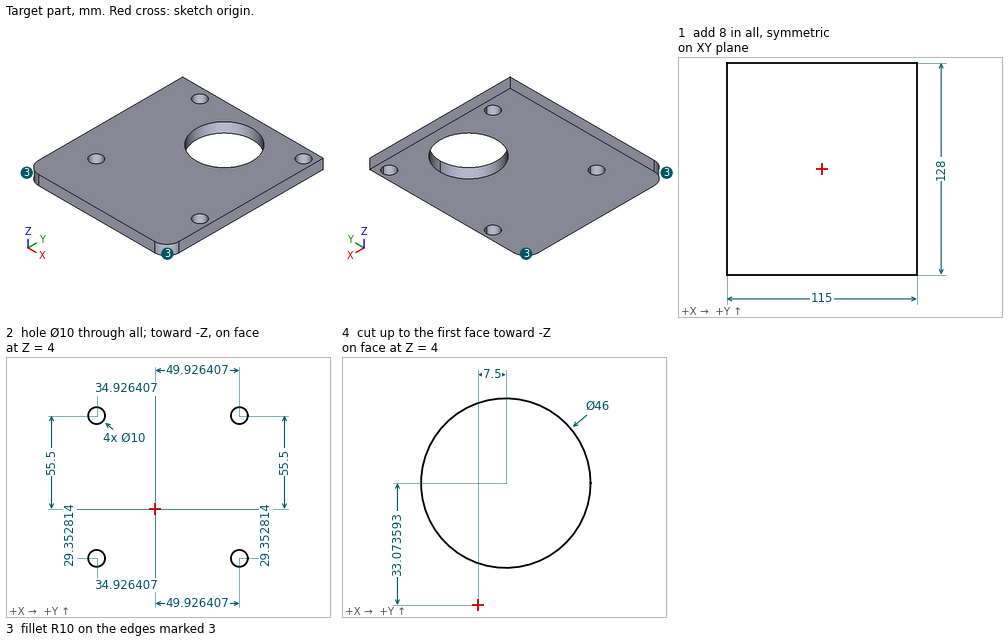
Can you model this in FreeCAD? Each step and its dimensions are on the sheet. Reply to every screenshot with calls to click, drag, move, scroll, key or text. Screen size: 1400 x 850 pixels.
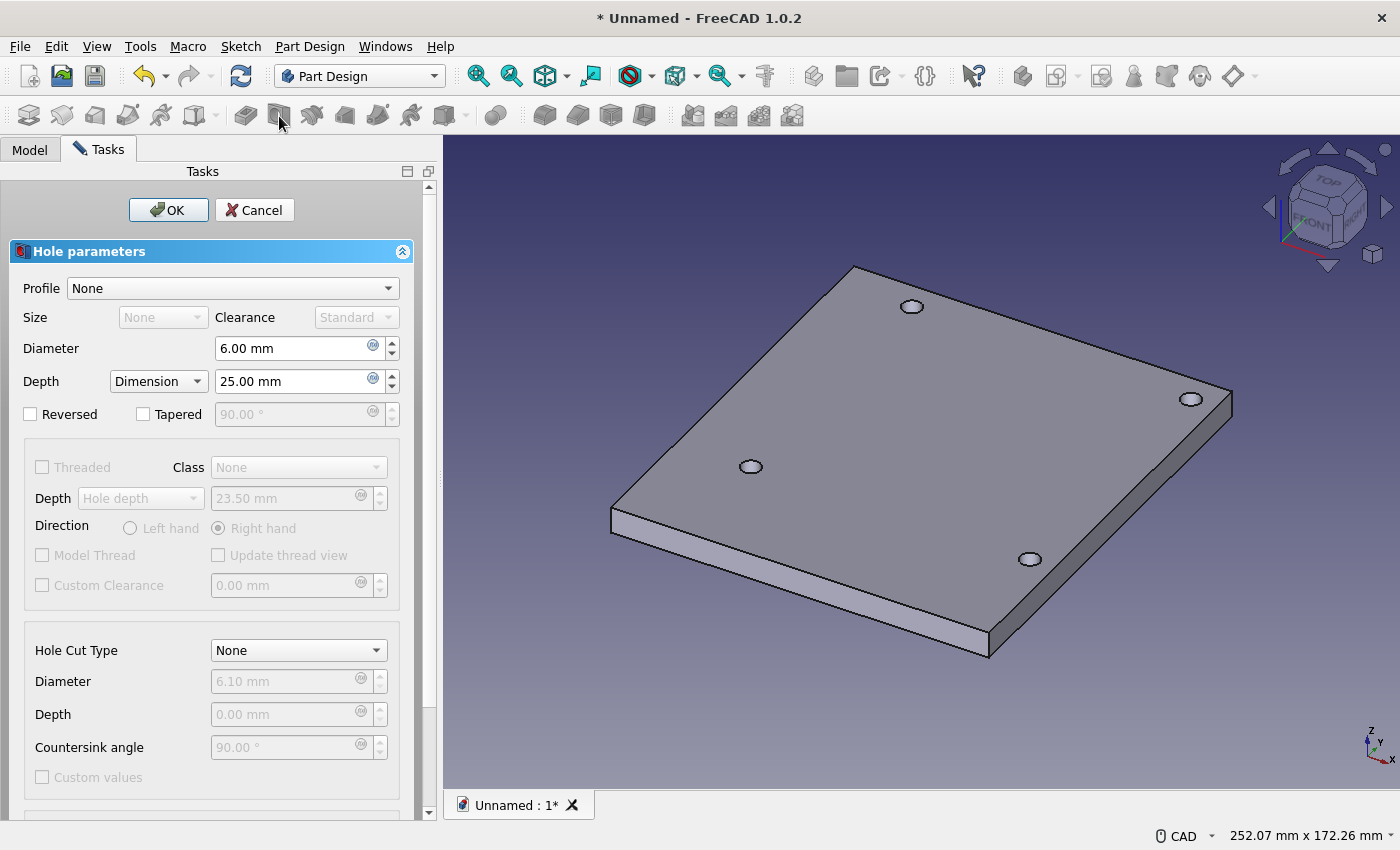
triple_click(300, 348)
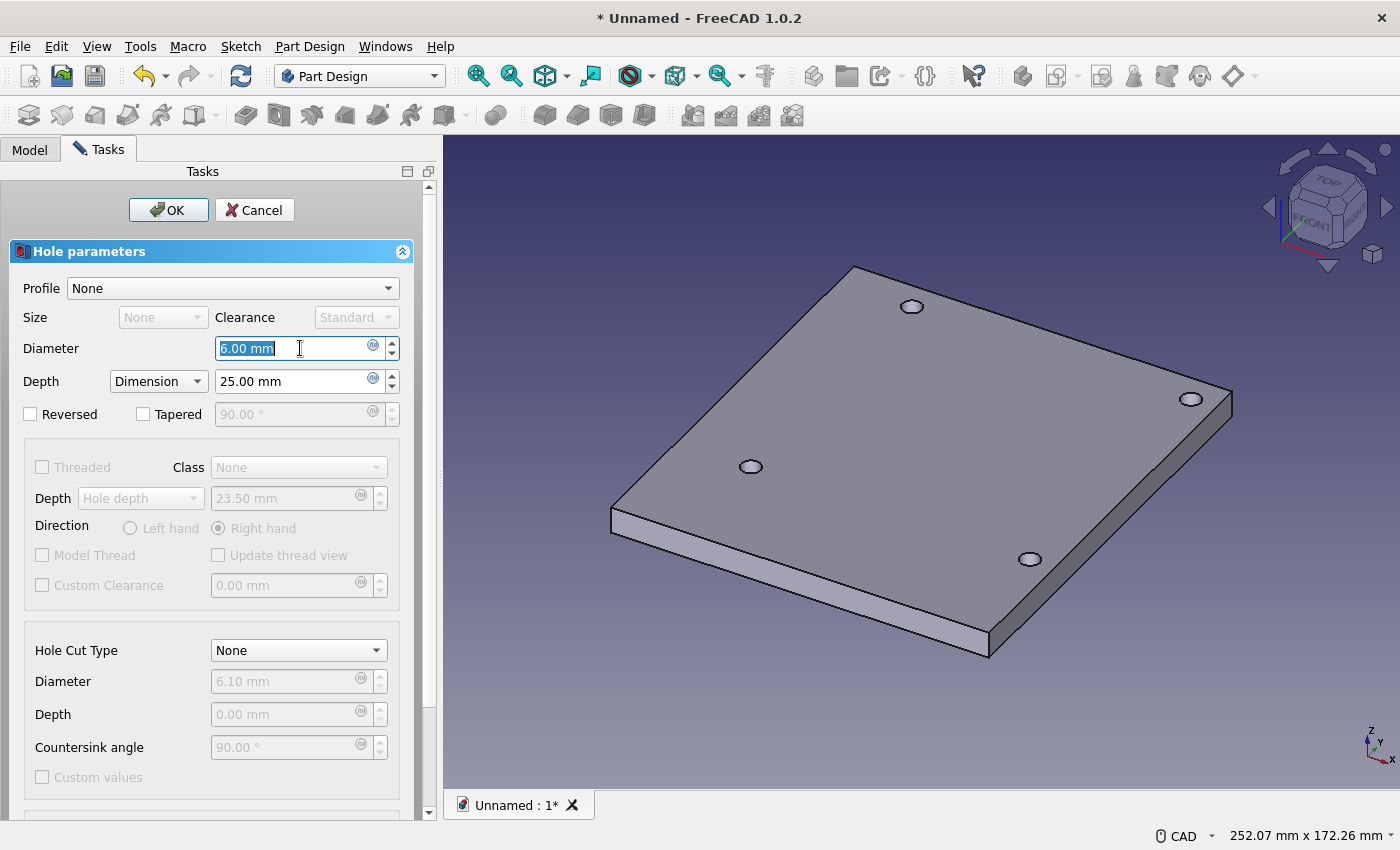
text(10)
key(Tab)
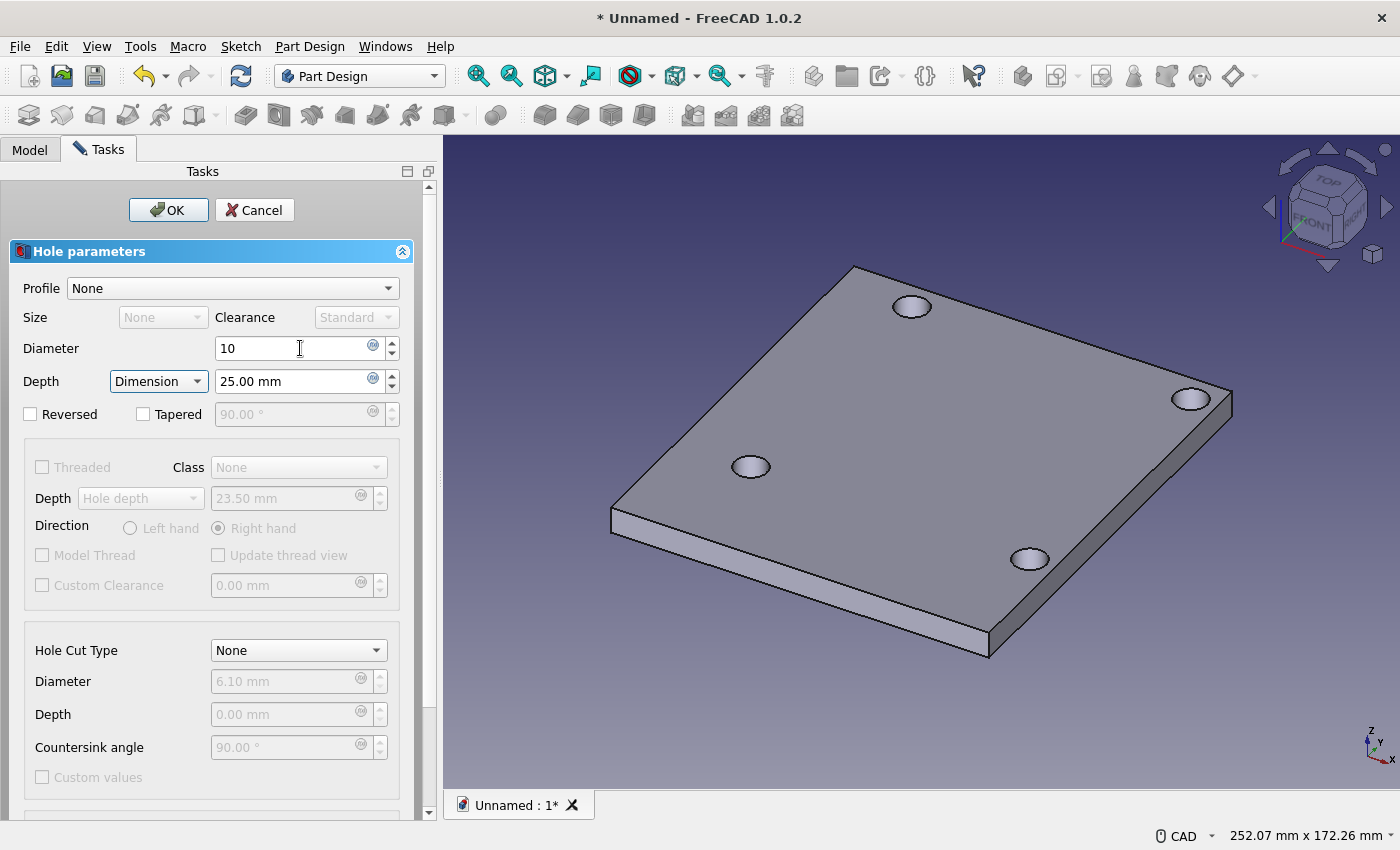
click(160, 382)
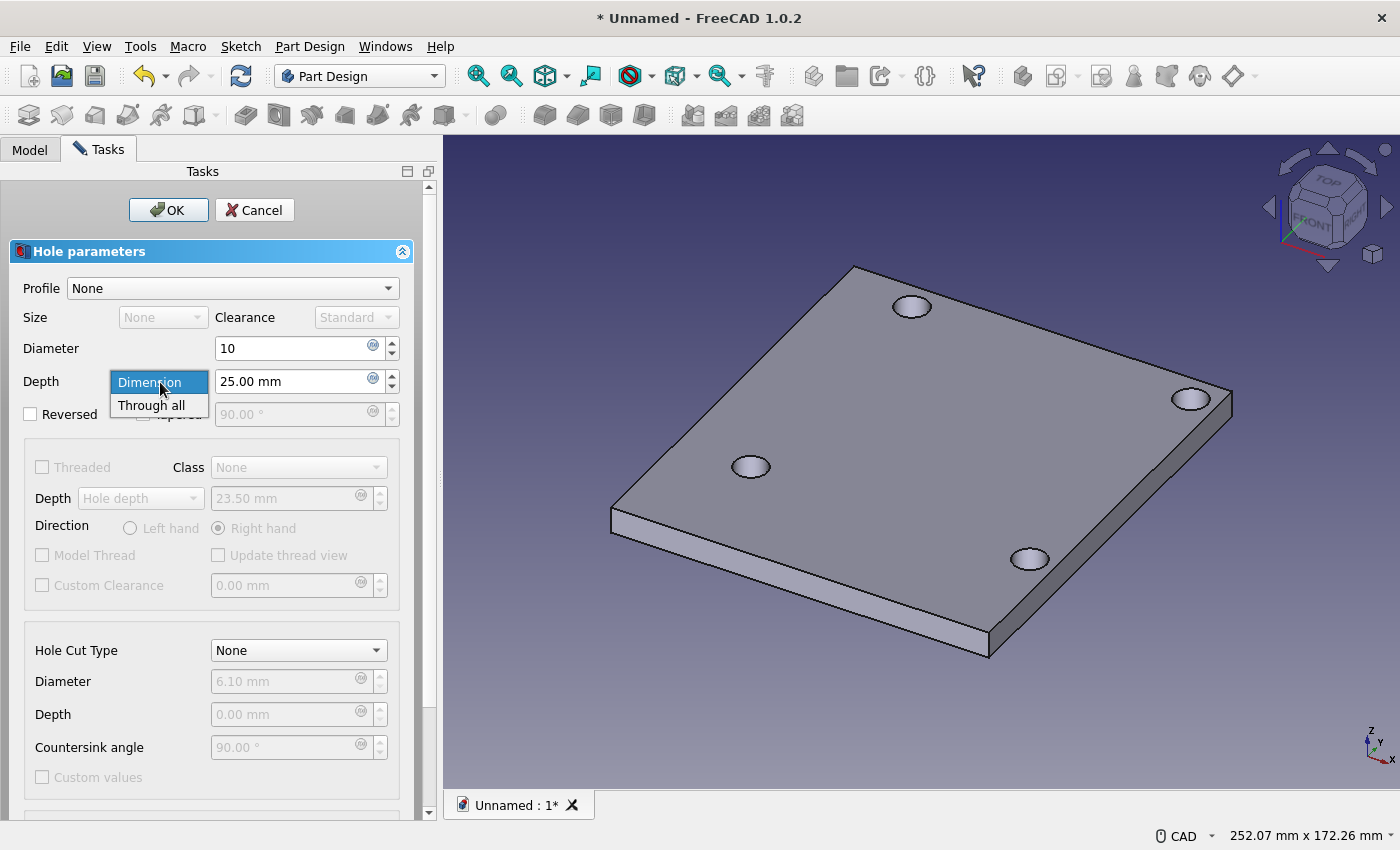
click(158, 406)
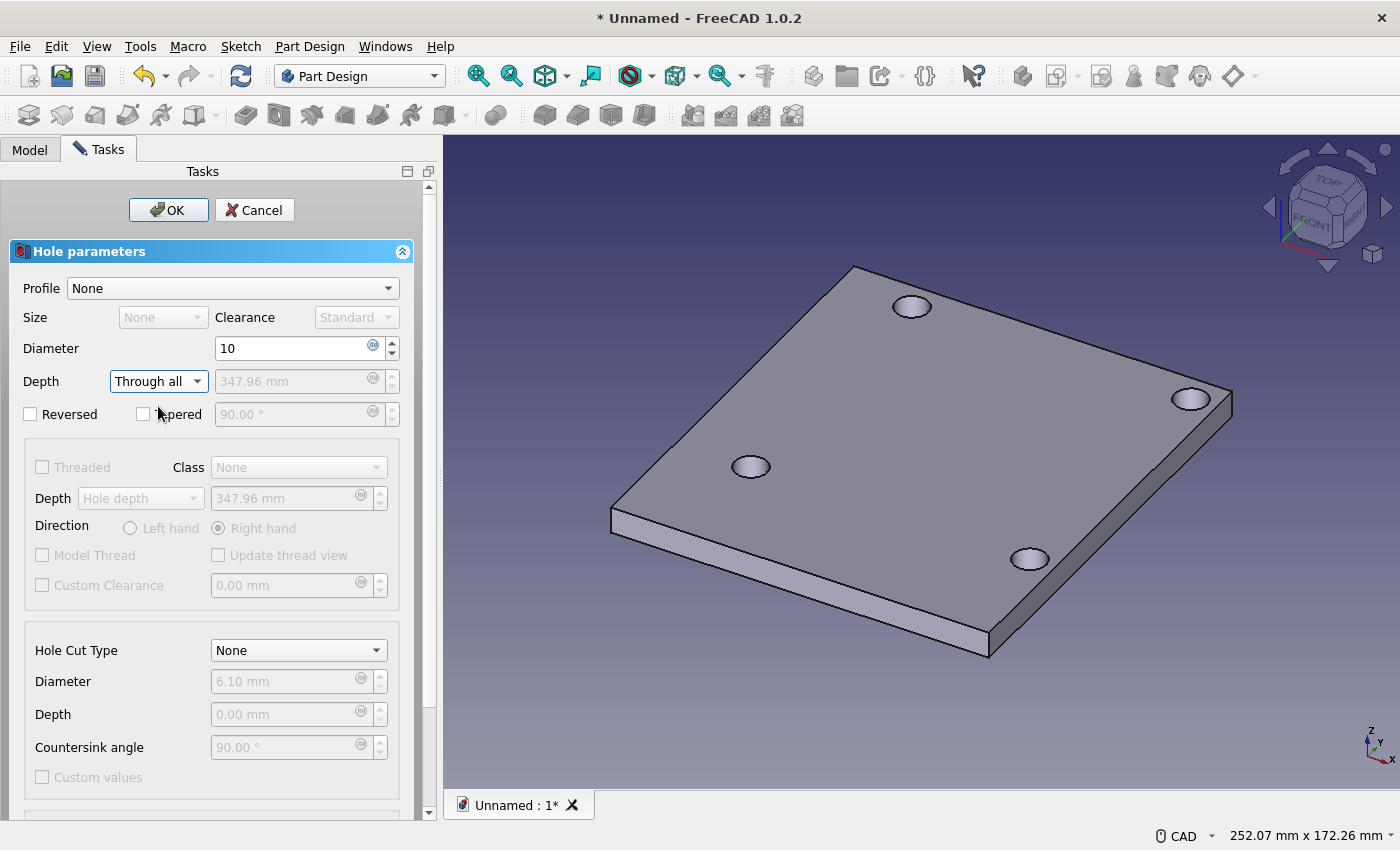
click(169, 210)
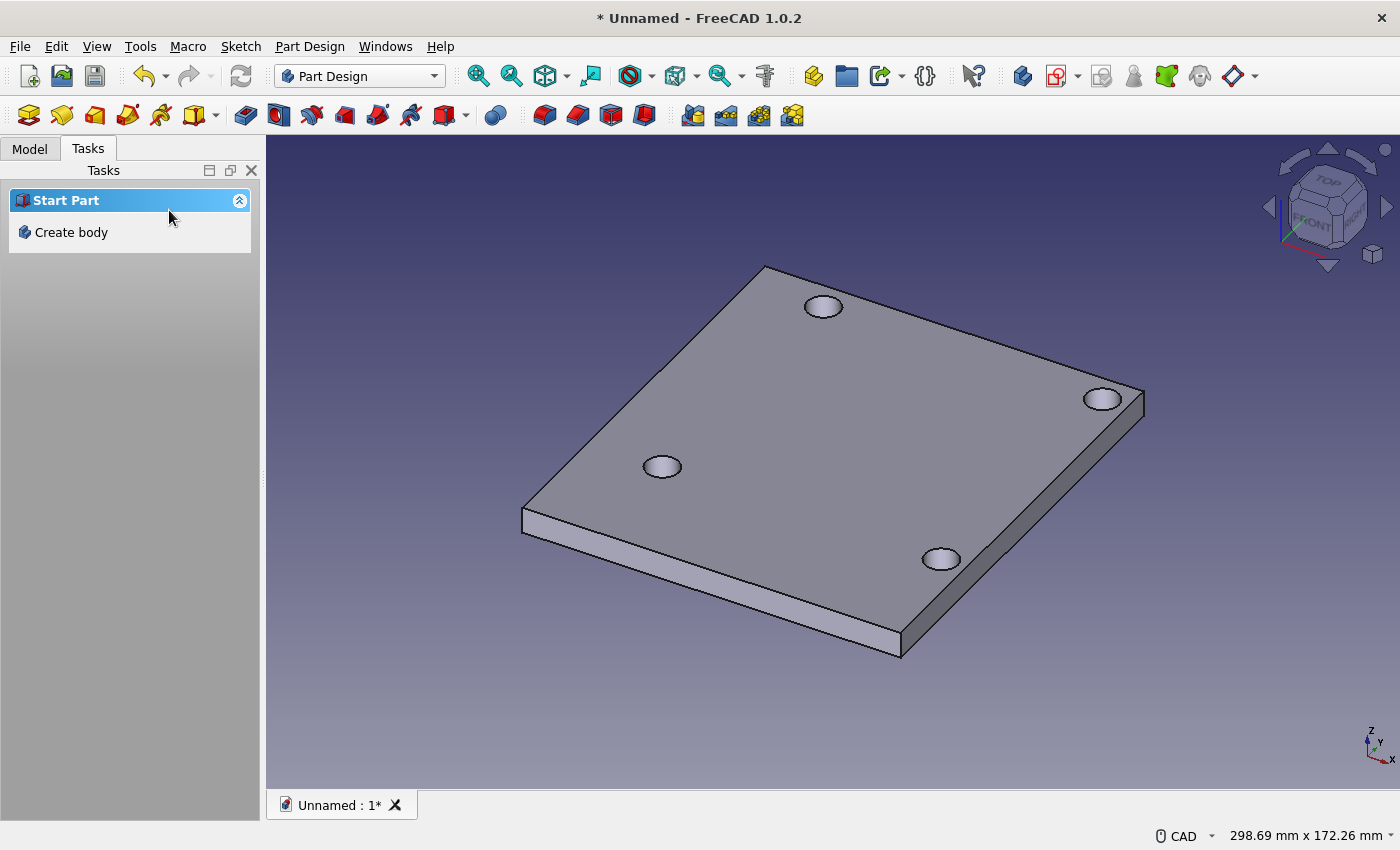
click(901, 644)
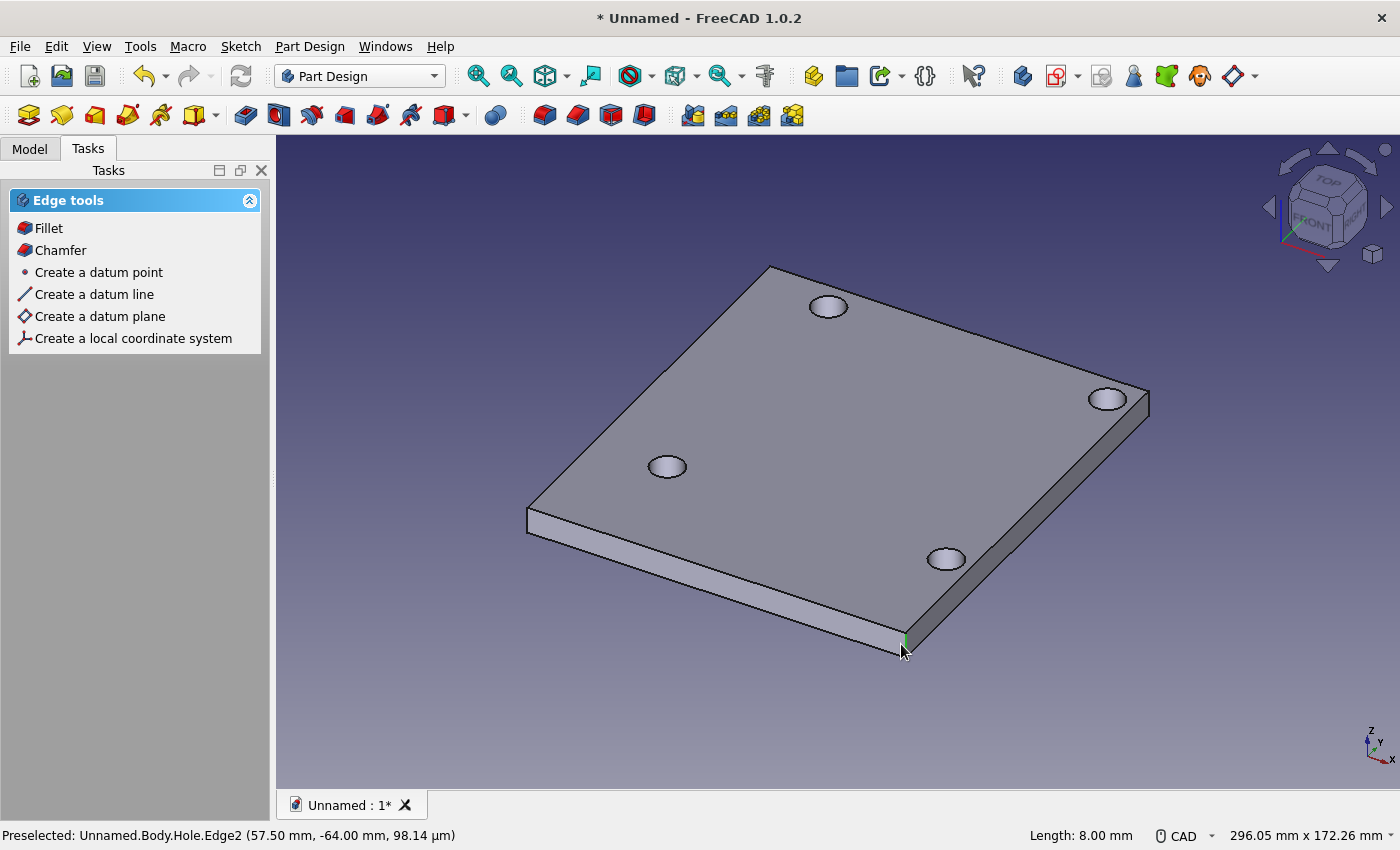
key(0)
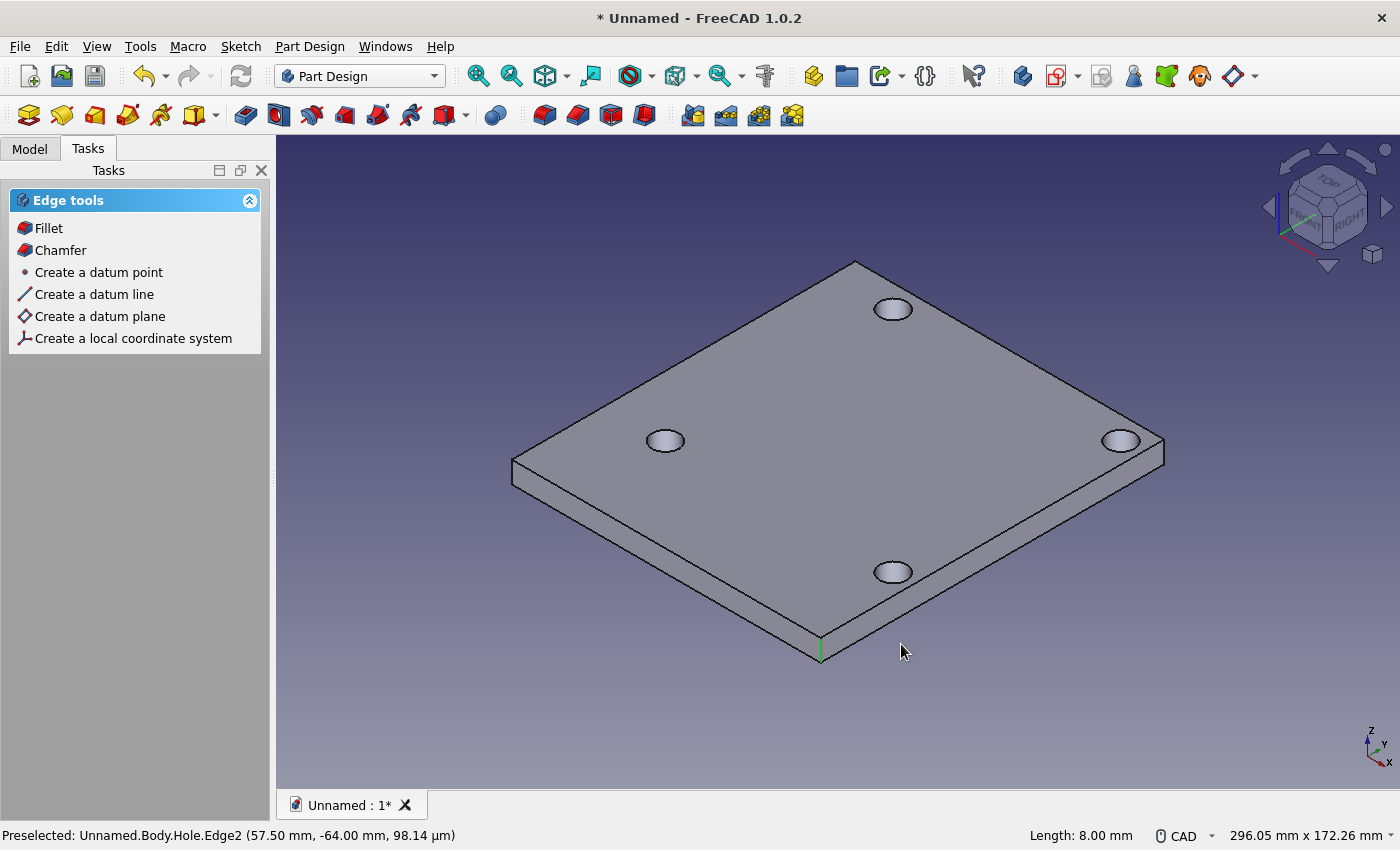
key(2)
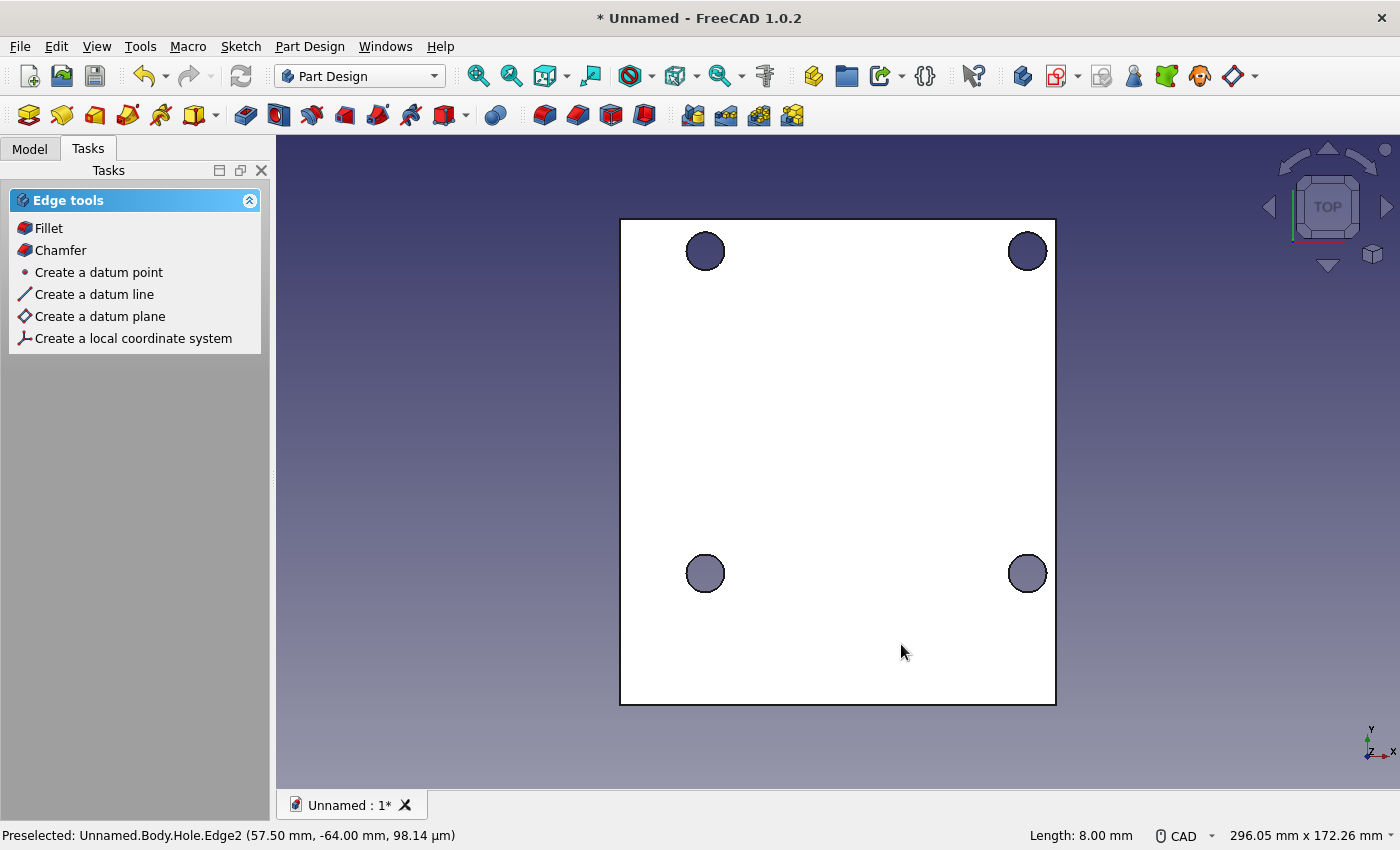
key(1)